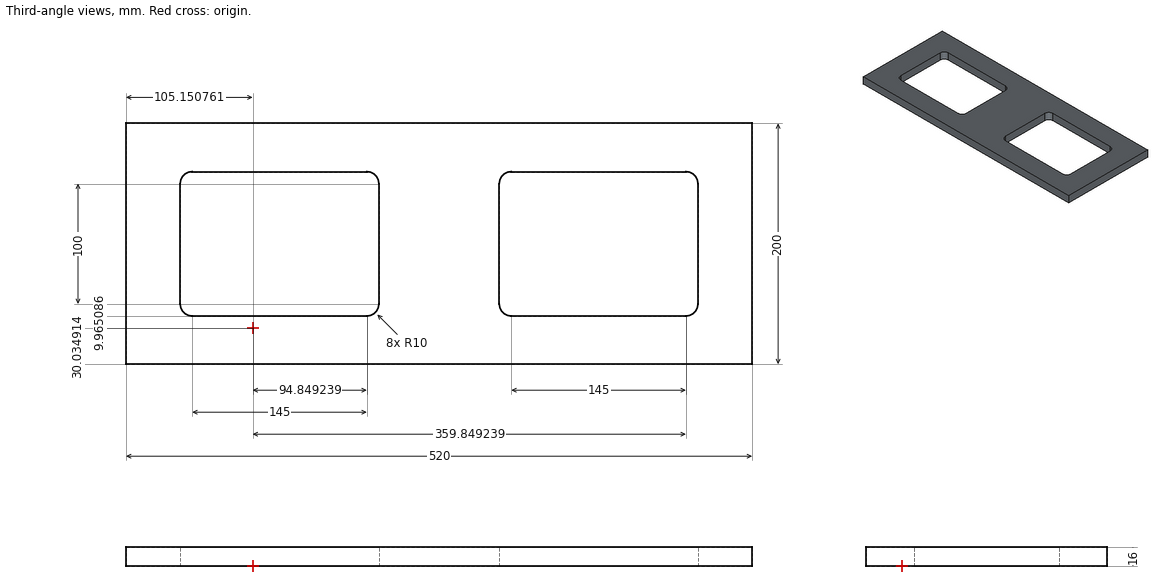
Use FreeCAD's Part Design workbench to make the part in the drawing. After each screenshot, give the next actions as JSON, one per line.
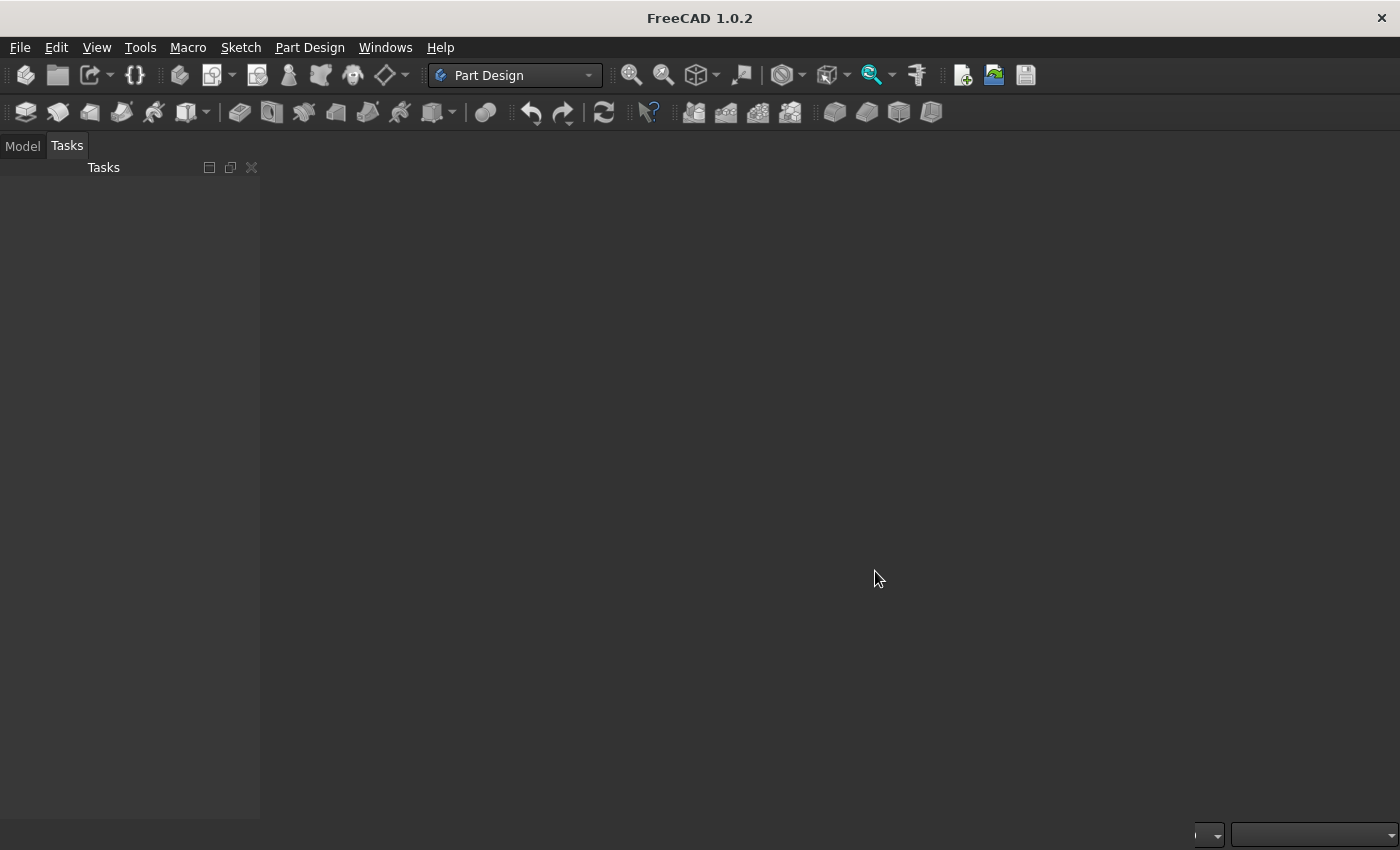
{"action": "key", "text": "ctrl+n"}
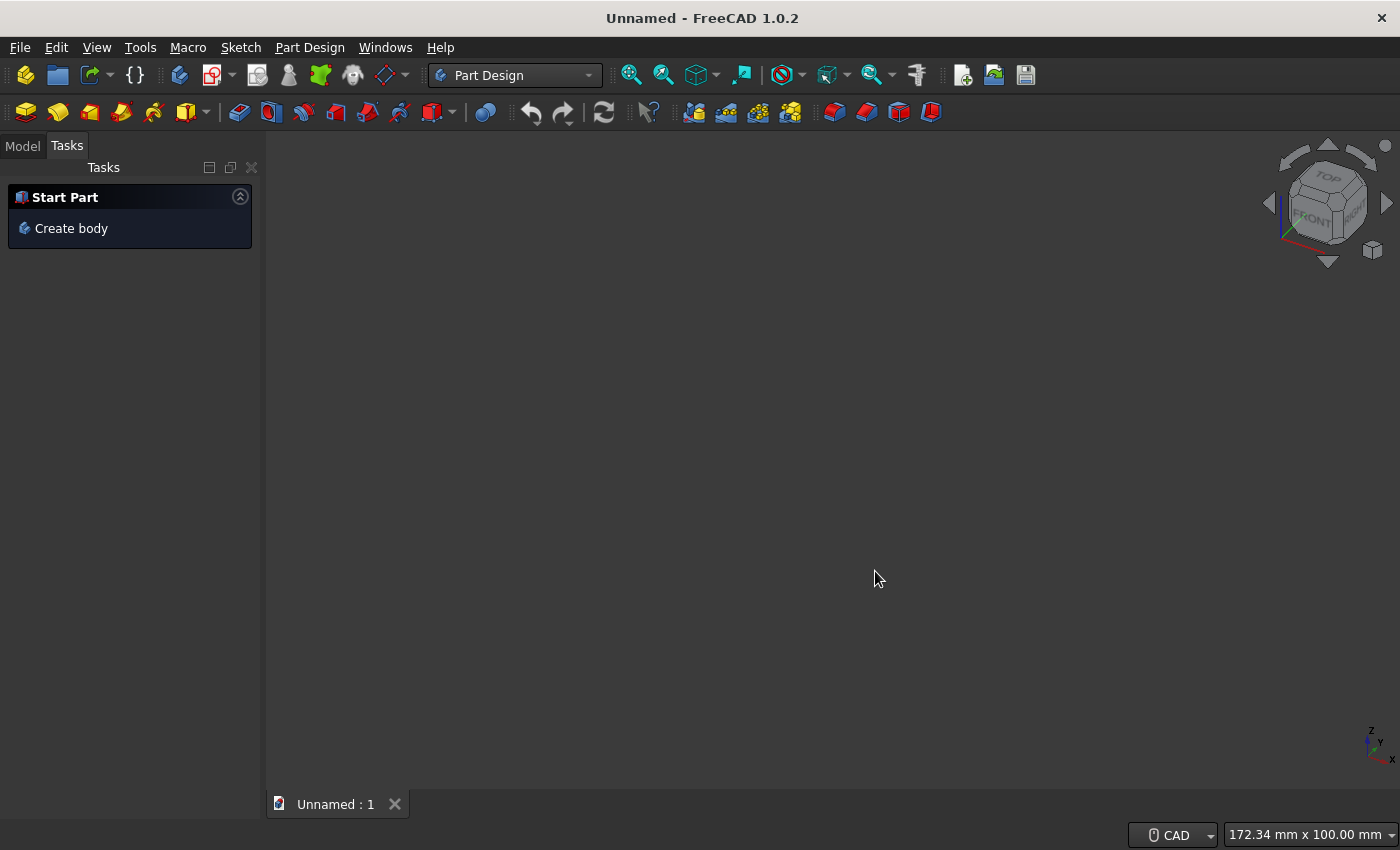
{"action": "left_click", "coordinate": [212, 76]}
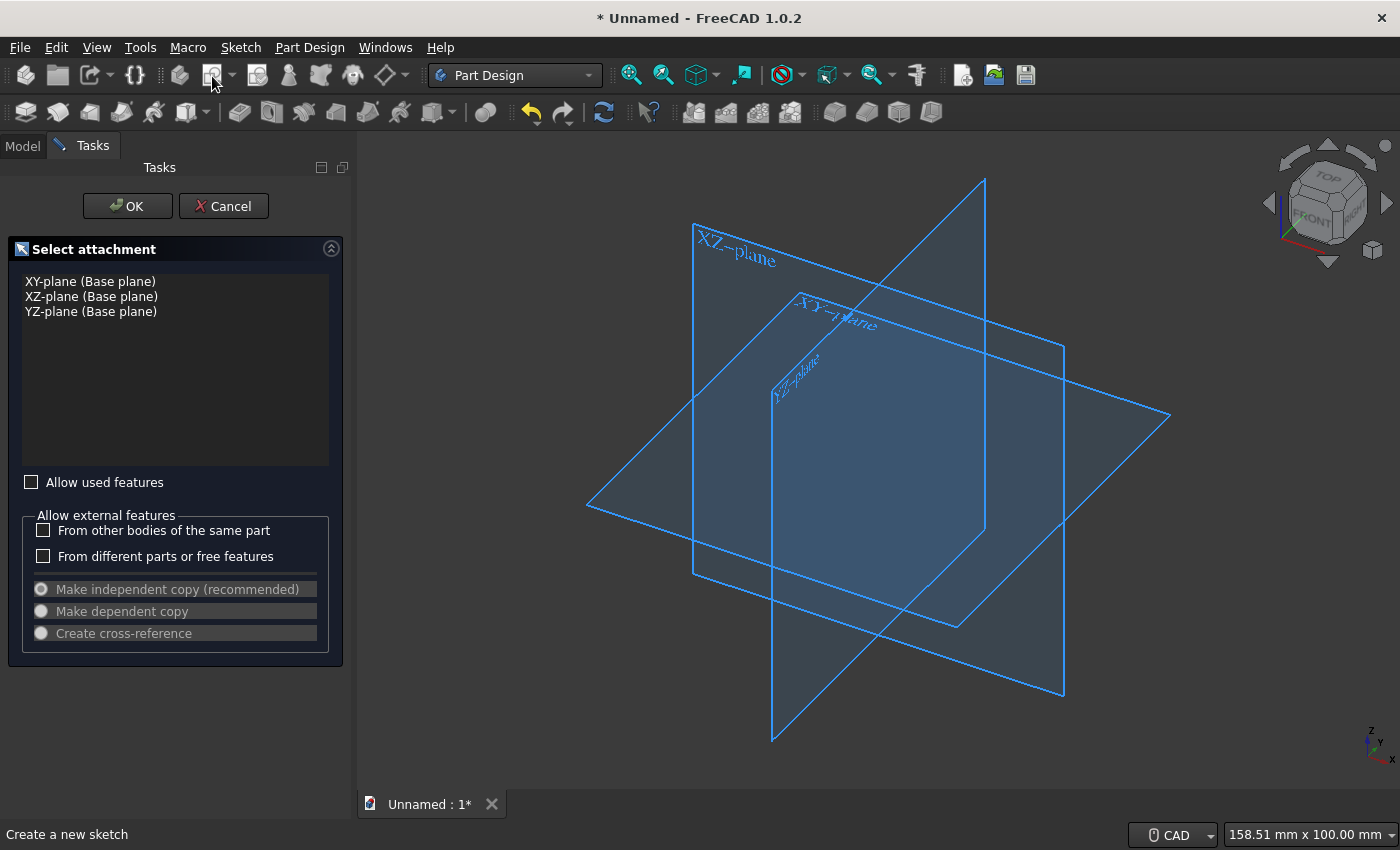
{"action": "left_click", "coordinate": [82, 282]}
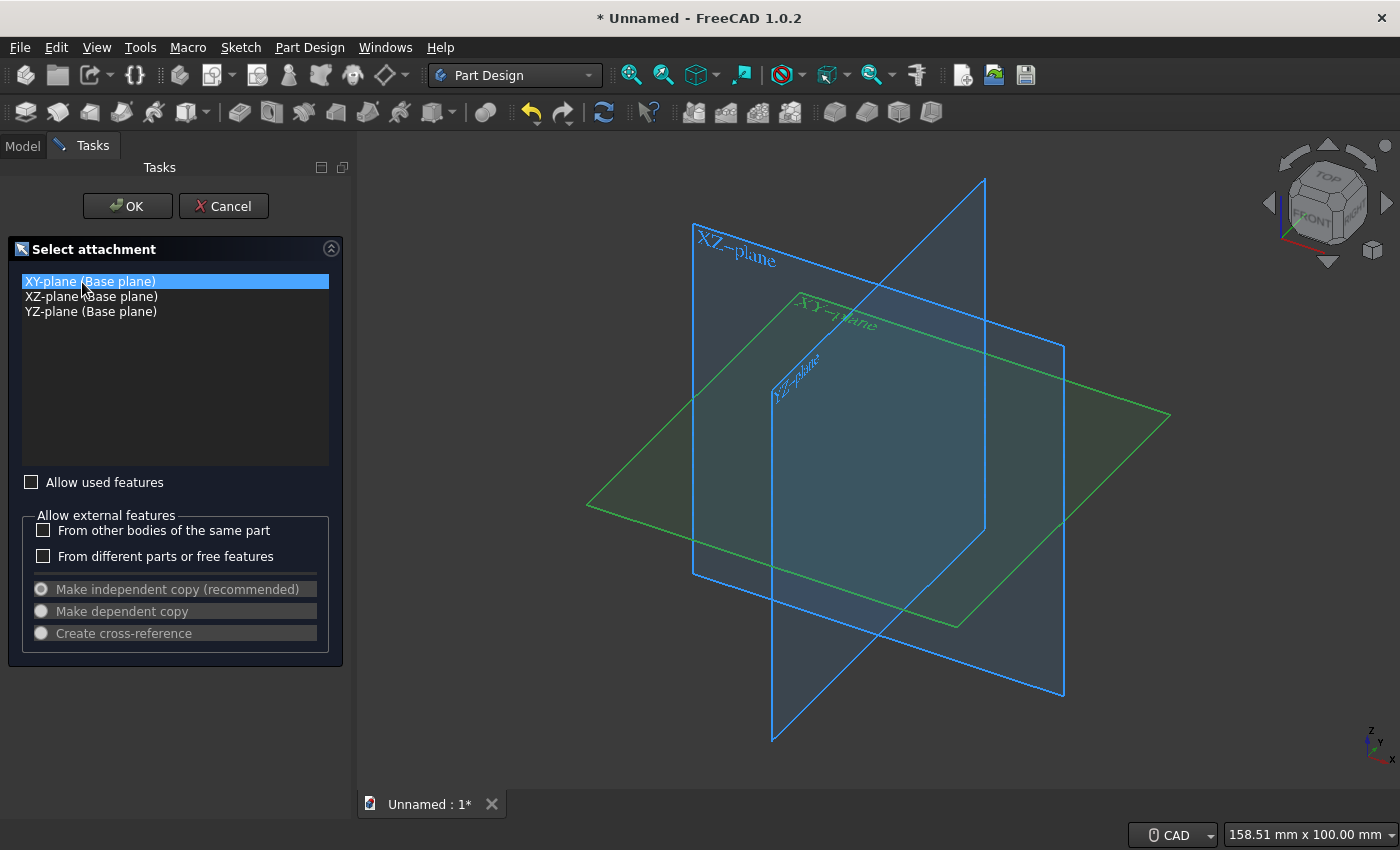
{"action": "left_click", "coordinate": [128, 206]}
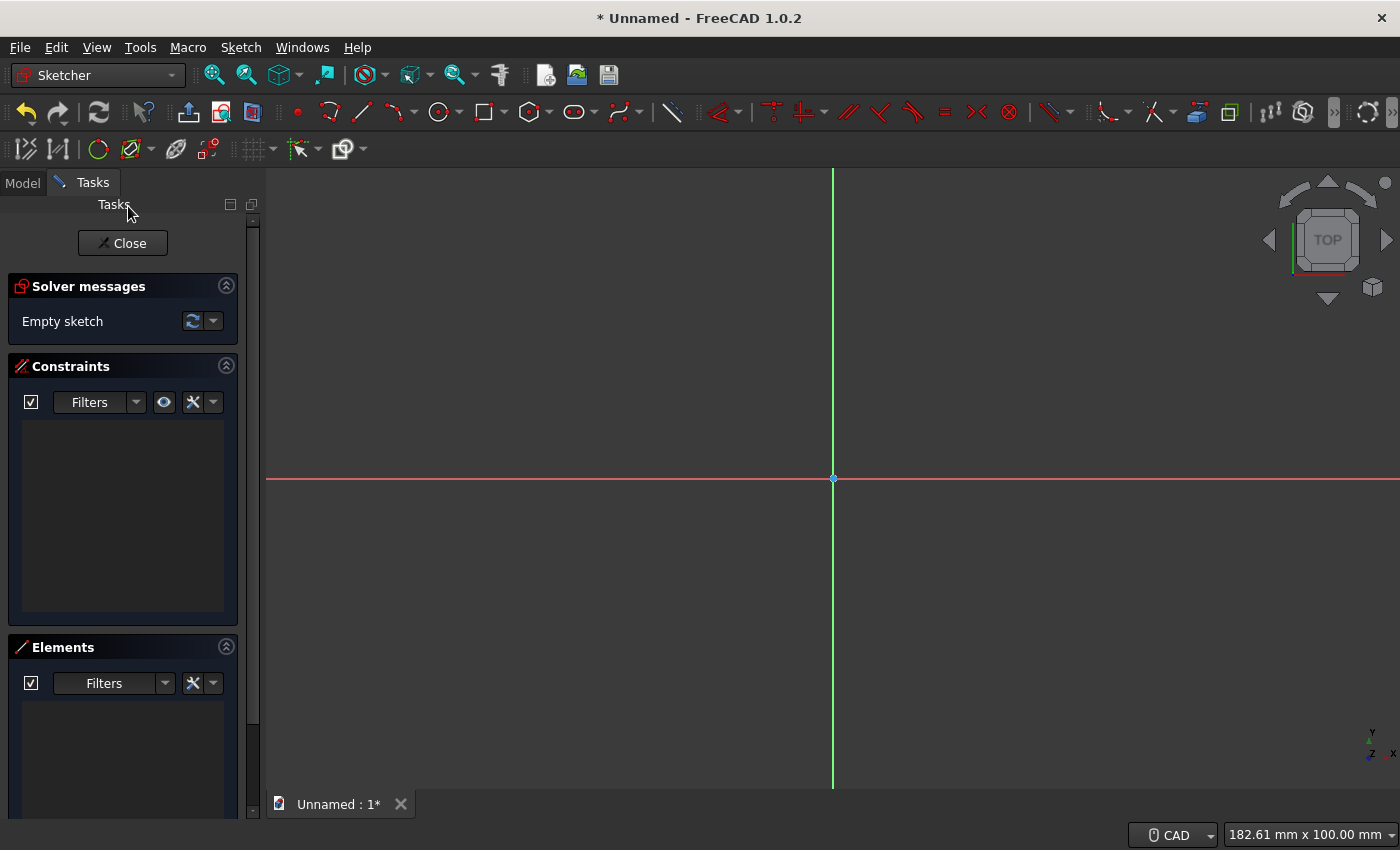
{"action": "scroll", "coordinate": [504, 588], "scroll_direction": "down", "scroll_amount": 8}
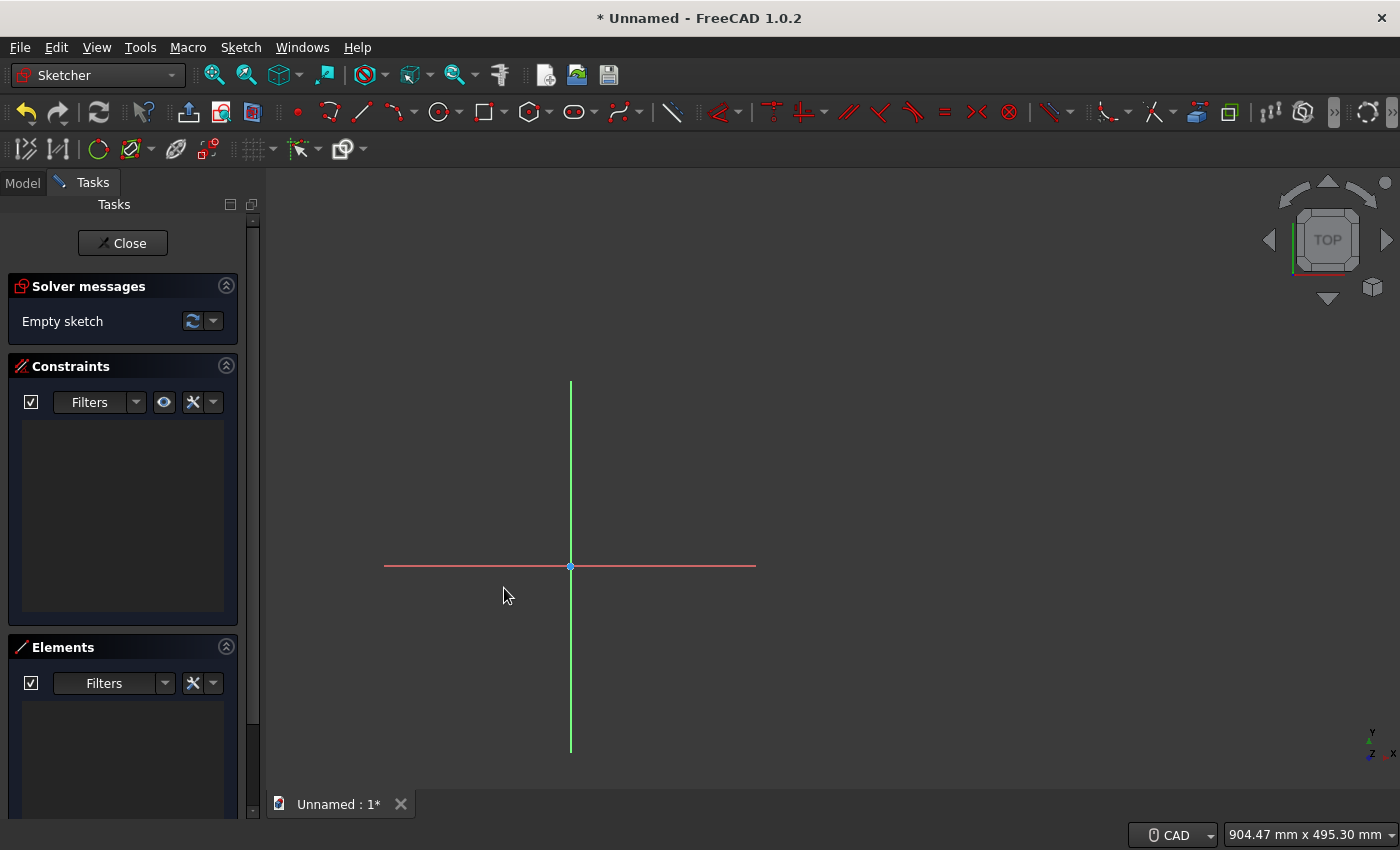
{"action": "left_click", "coordinate": [484, 112]}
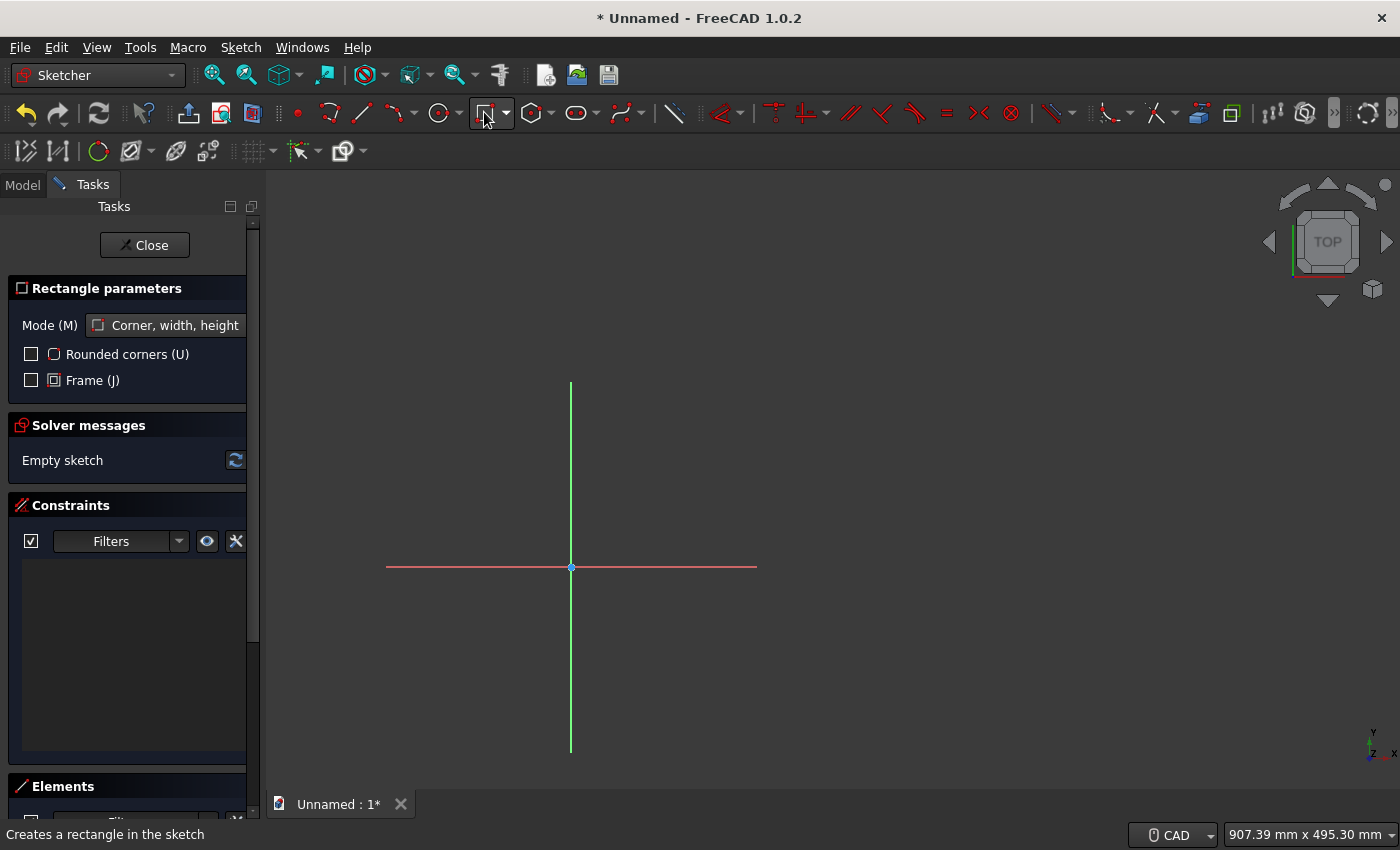
{"action": "left_click", "coordinate": [440, 355]}
{"action": "mouse_move", "coordinate": [1090, 605]}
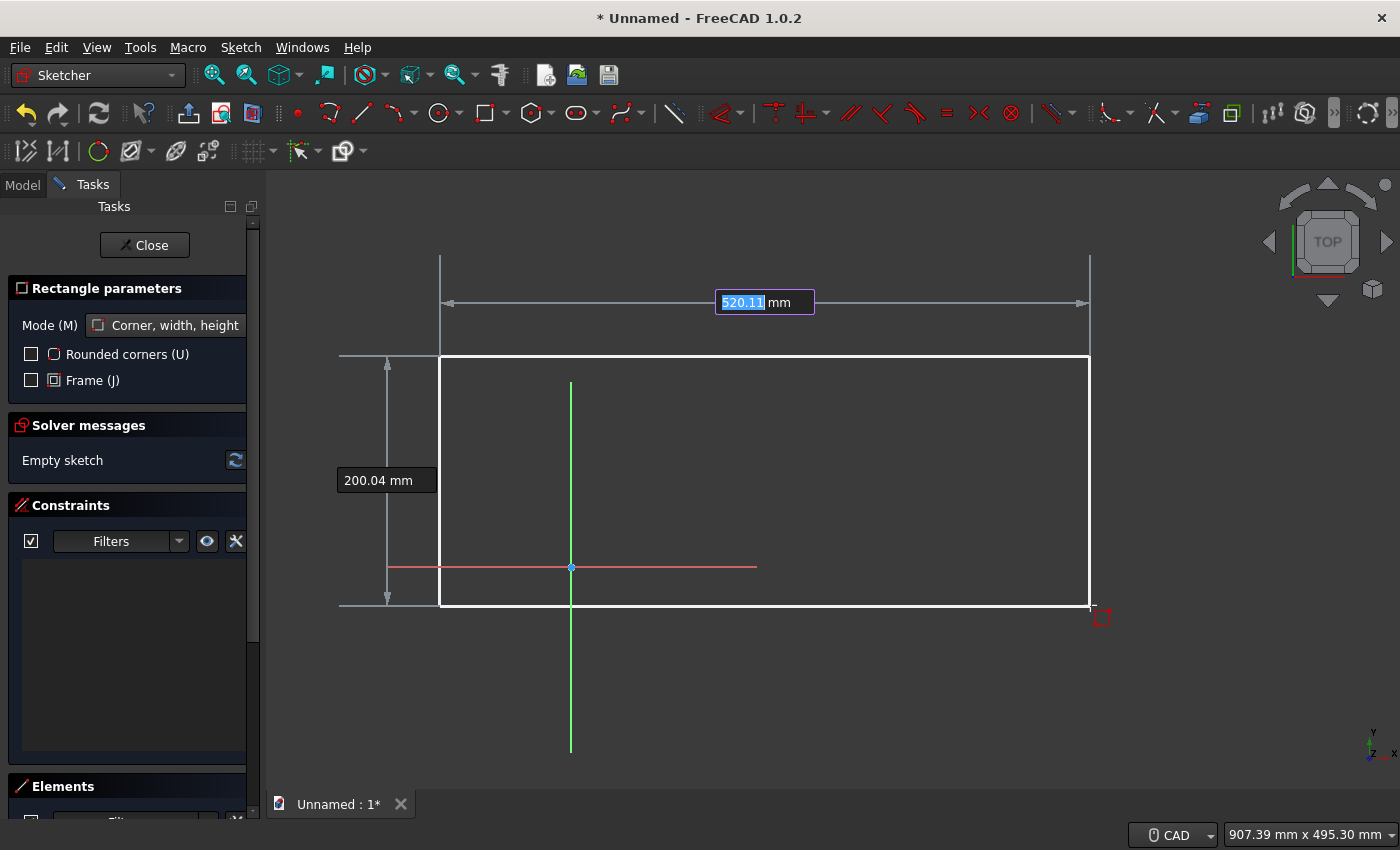
{"action": "type", "text": "520"}
{"action": "key", "text": "Tab"}
{"action": "type", "text": "200"}
{"action": "key", "text": "Return"}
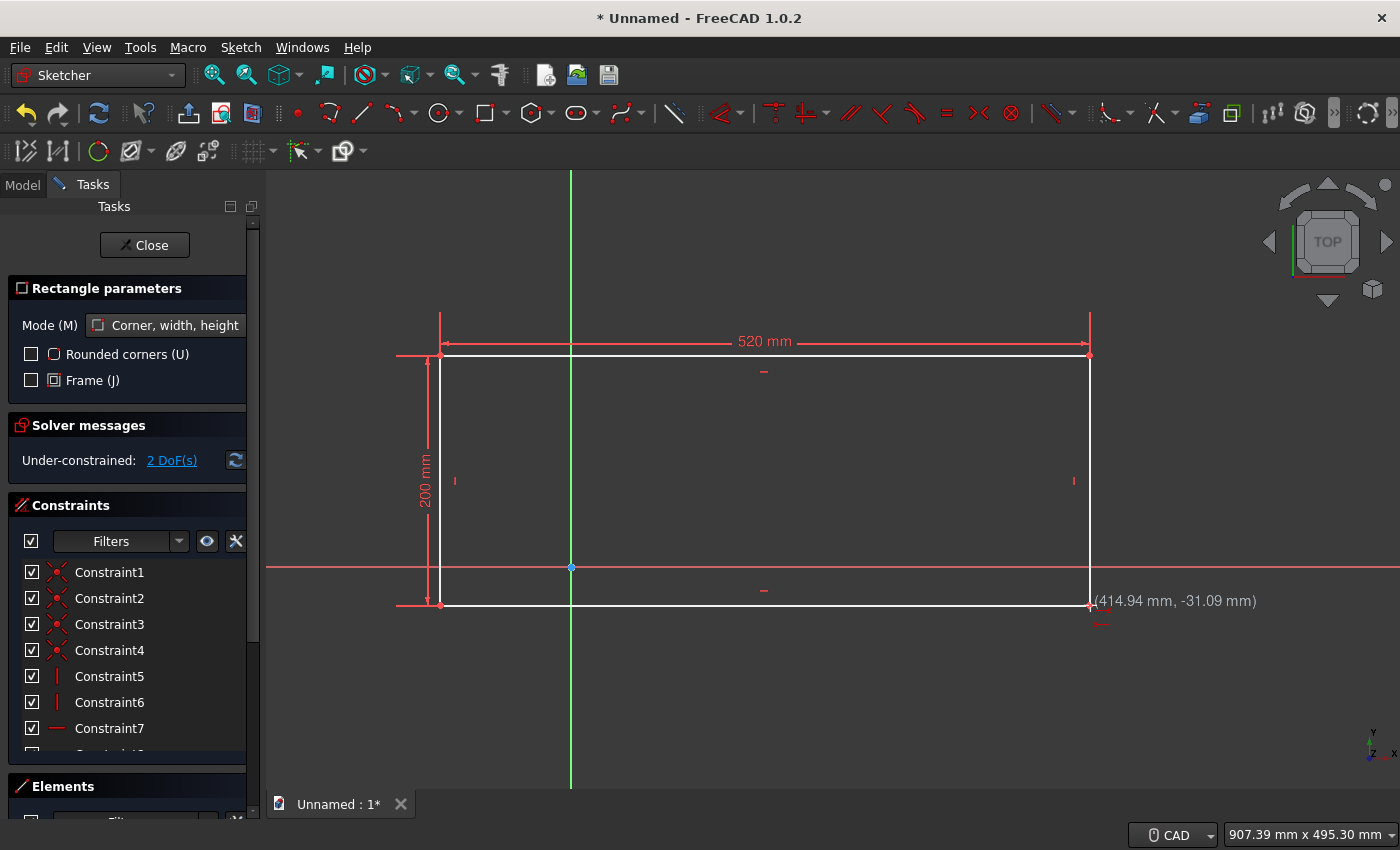
{"action": "key", "text": "g l"}